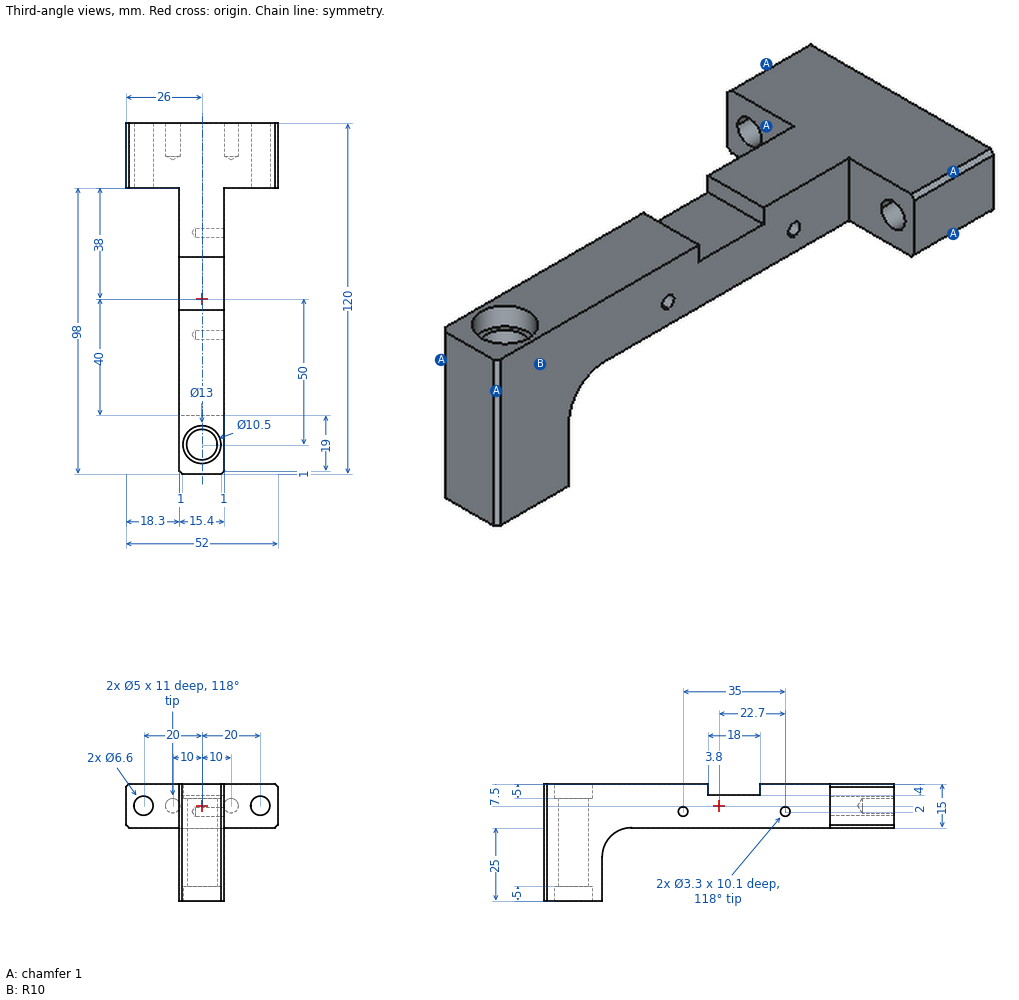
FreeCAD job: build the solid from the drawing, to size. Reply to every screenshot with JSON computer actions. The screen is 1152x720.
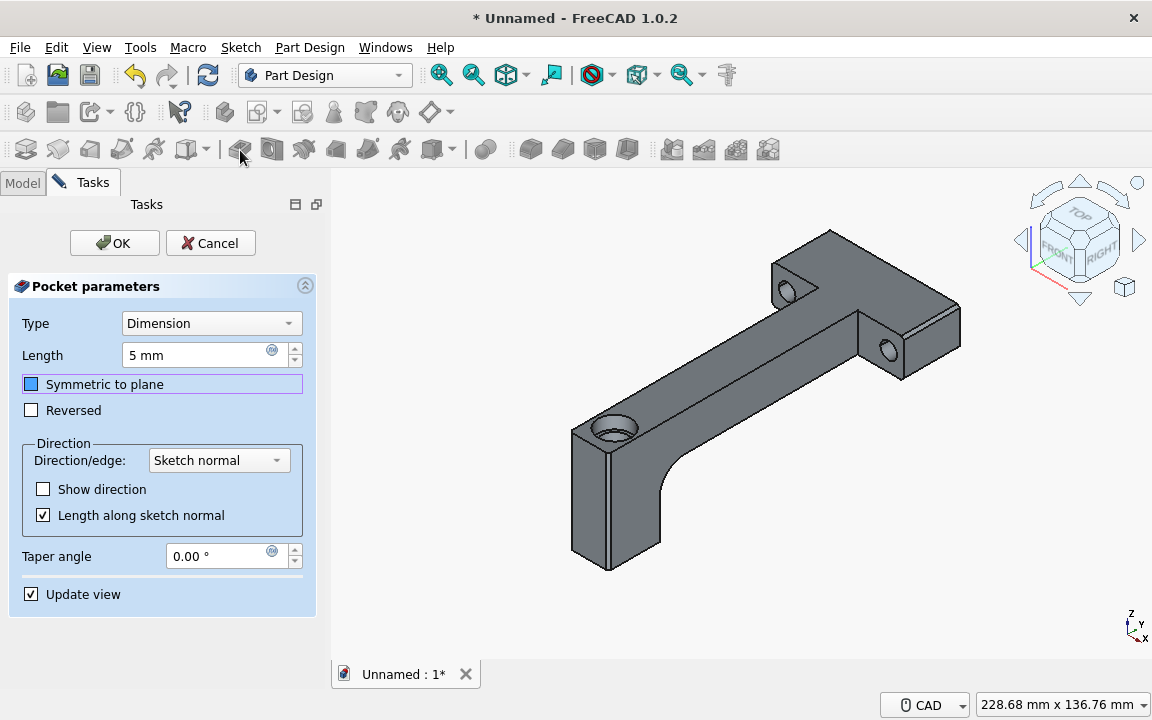
{"action": "left_click", "coordinate": [115, 243]}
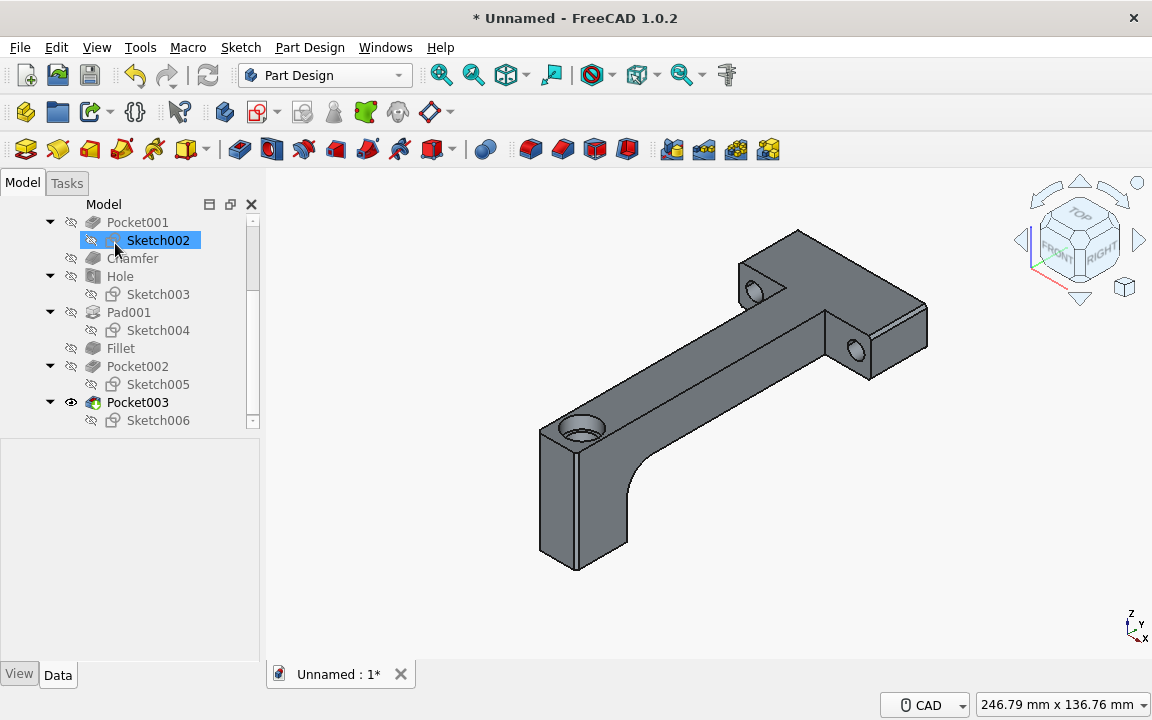
{"action": "scroll", "coordinate": [140, 326], "scroll_direction": "down", "scroll_amount": 3}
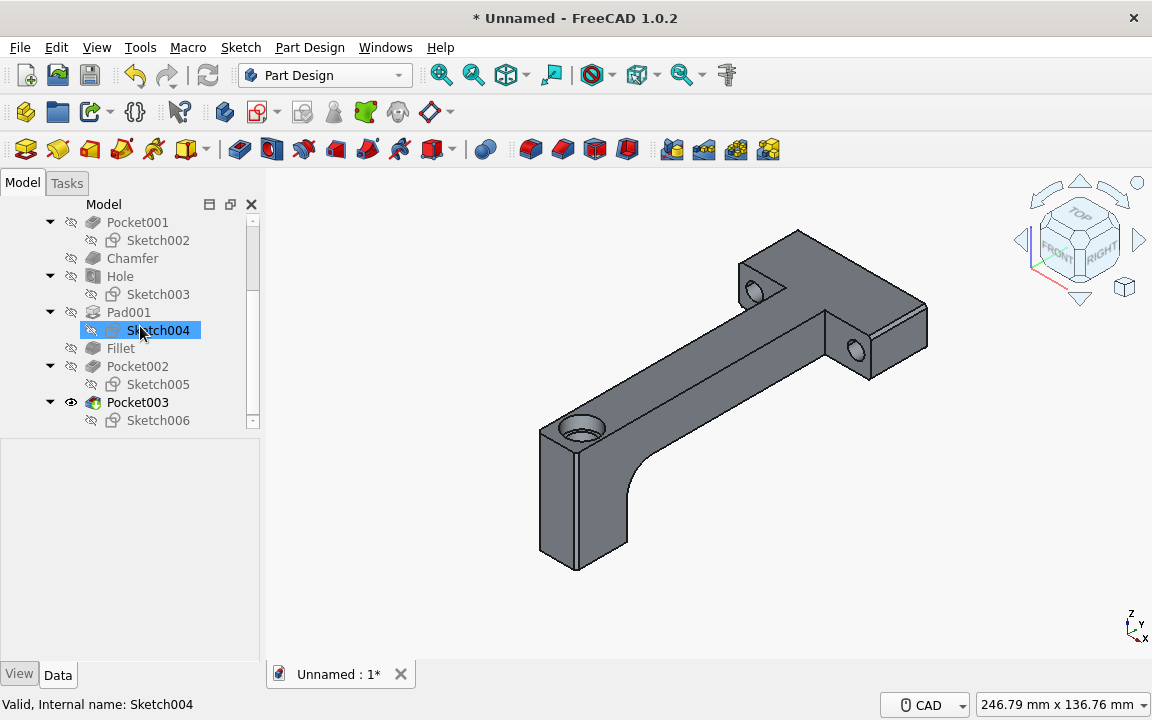
{"action": "scroll", "coordinate": [140, 326], "scroll_direction": "up", "scroll_amount": 15}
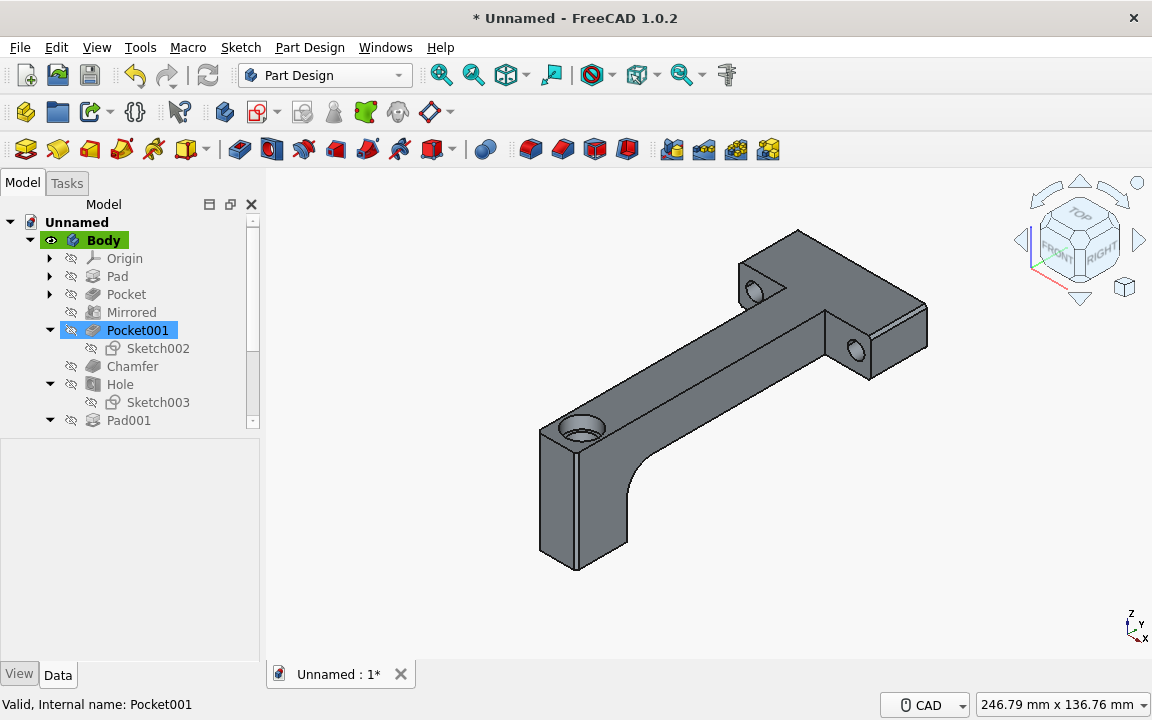
{"action": "left_click", "coordinate": [50, 258]}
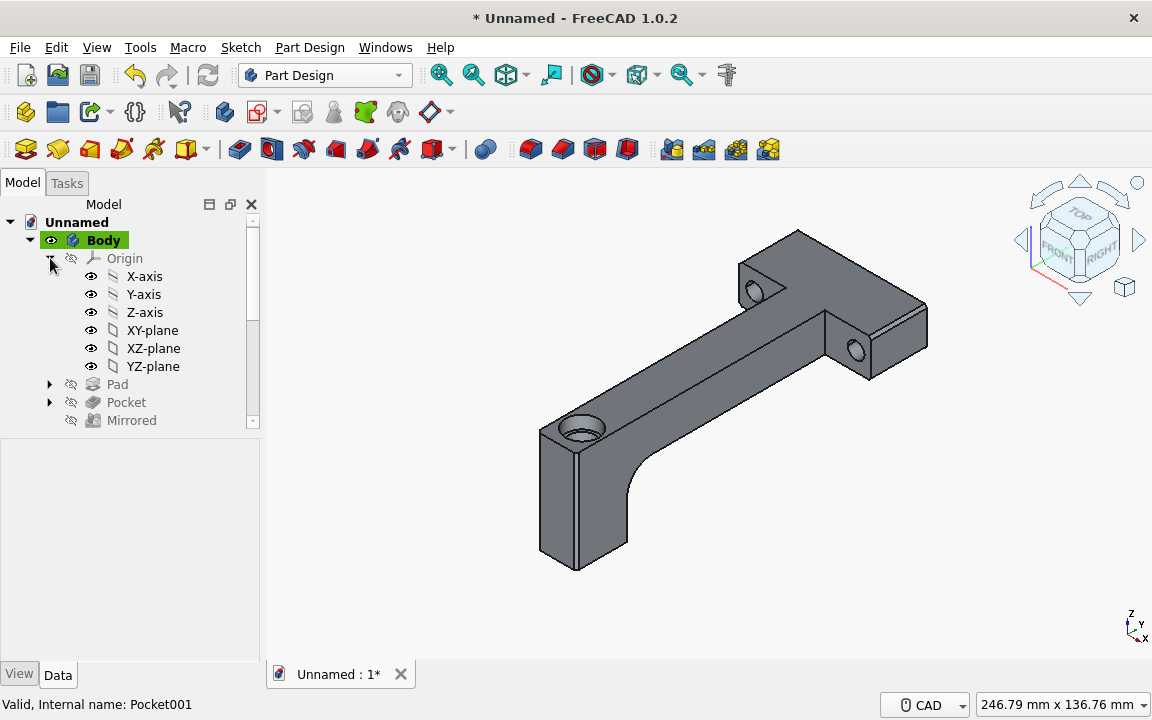
{"action": "left_click", "coordinate": [136, 330]}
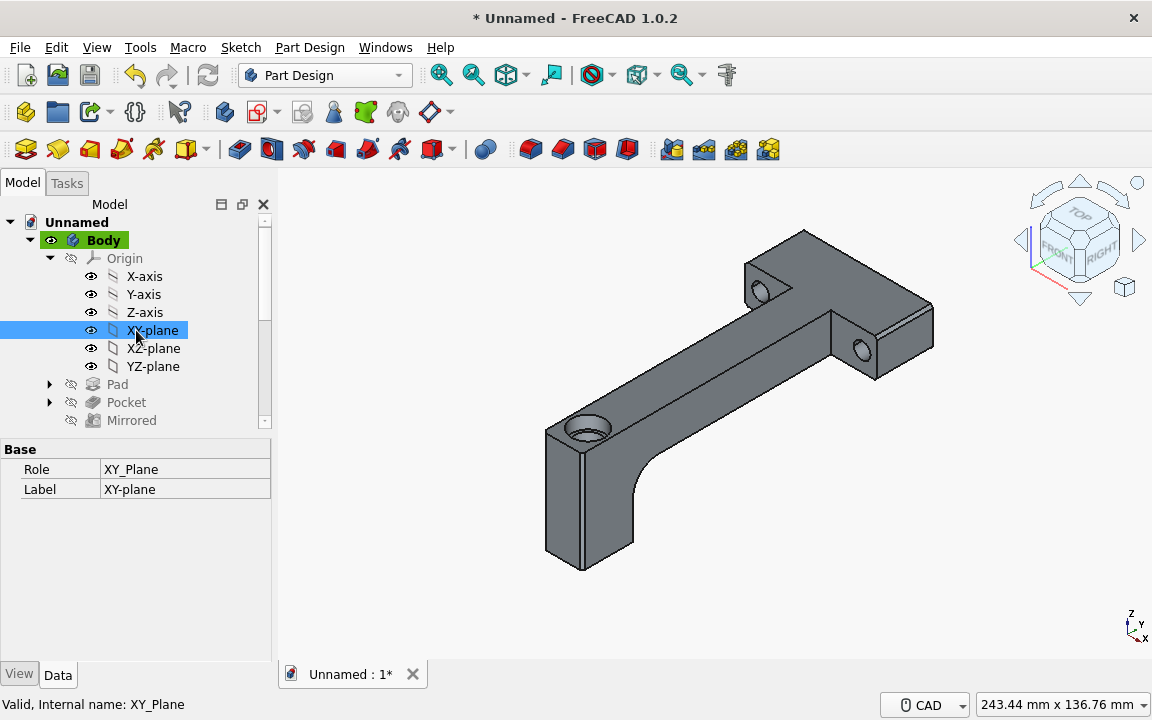
{"action": "left_click", "coordinate": [430, 112]}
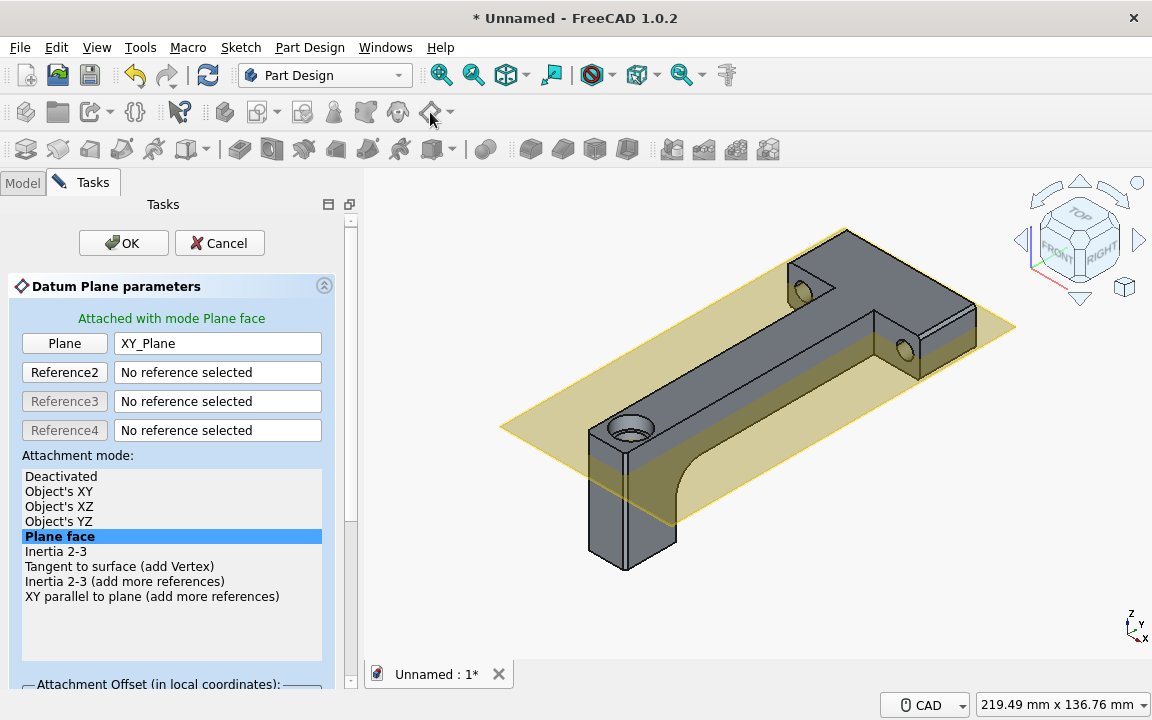
{"action": "scroll", "coordinate": [351, 451], "scroll_direction": "down", "scroll_amount": 3}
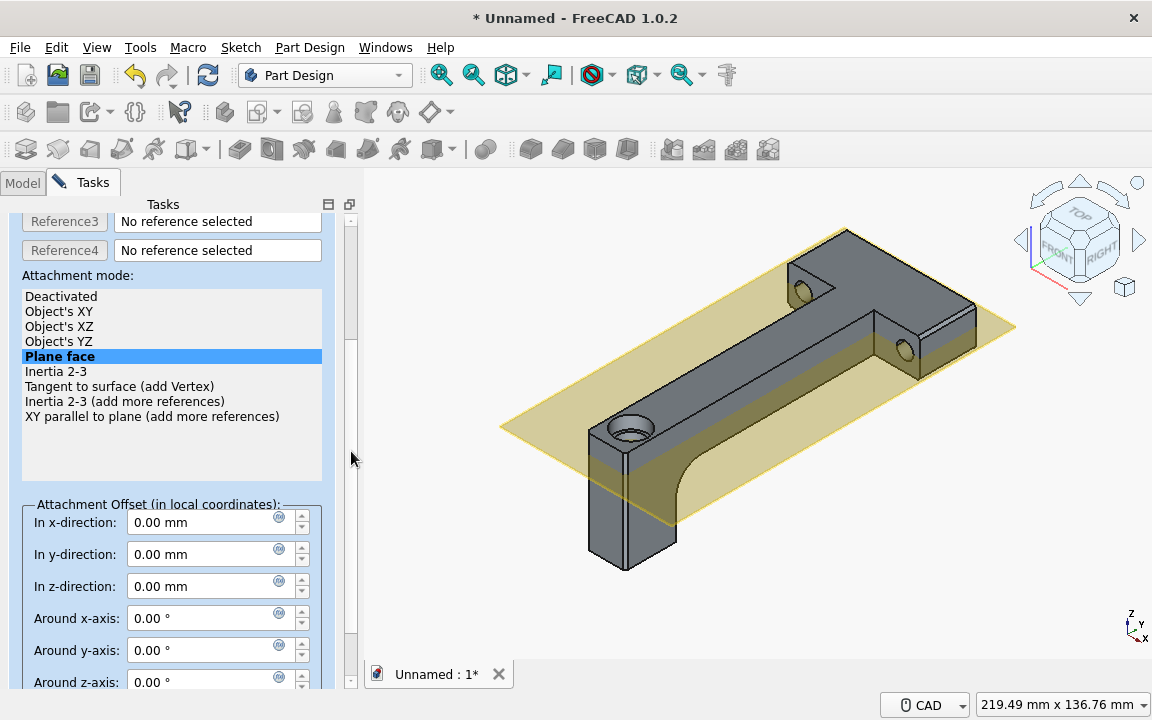
{"action": "triple_click", "coordinate": [210, 586]}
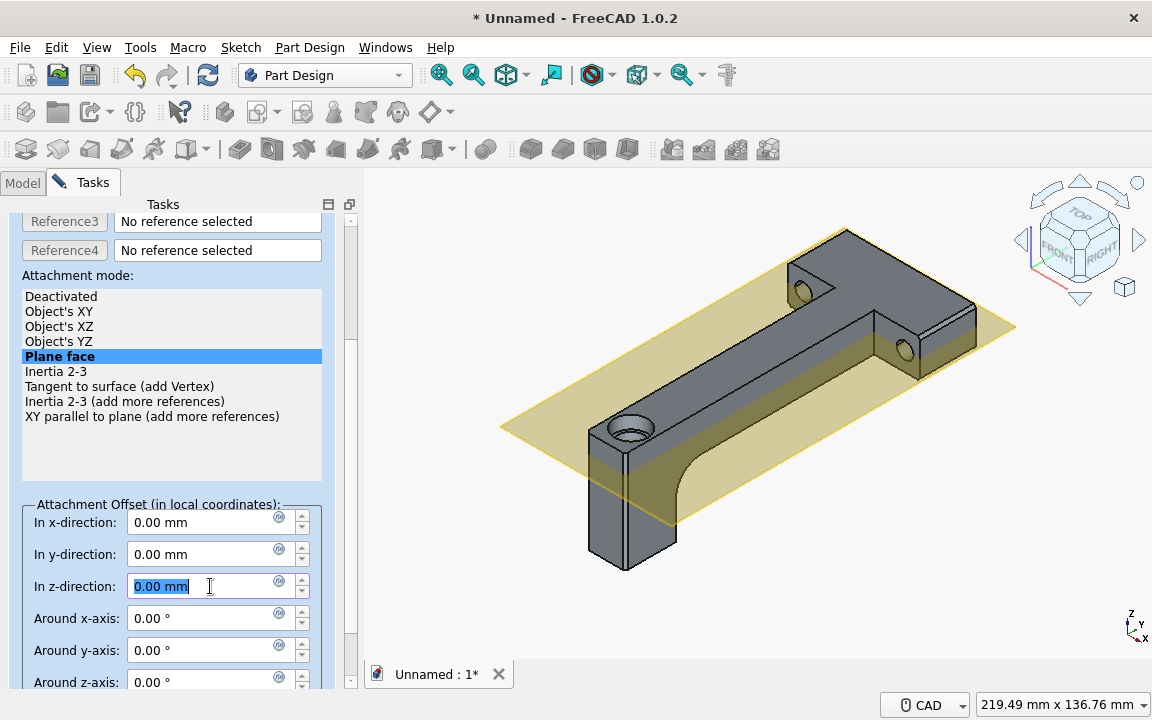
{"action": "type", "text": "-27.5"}
{"action": "key", "text": "Tab"}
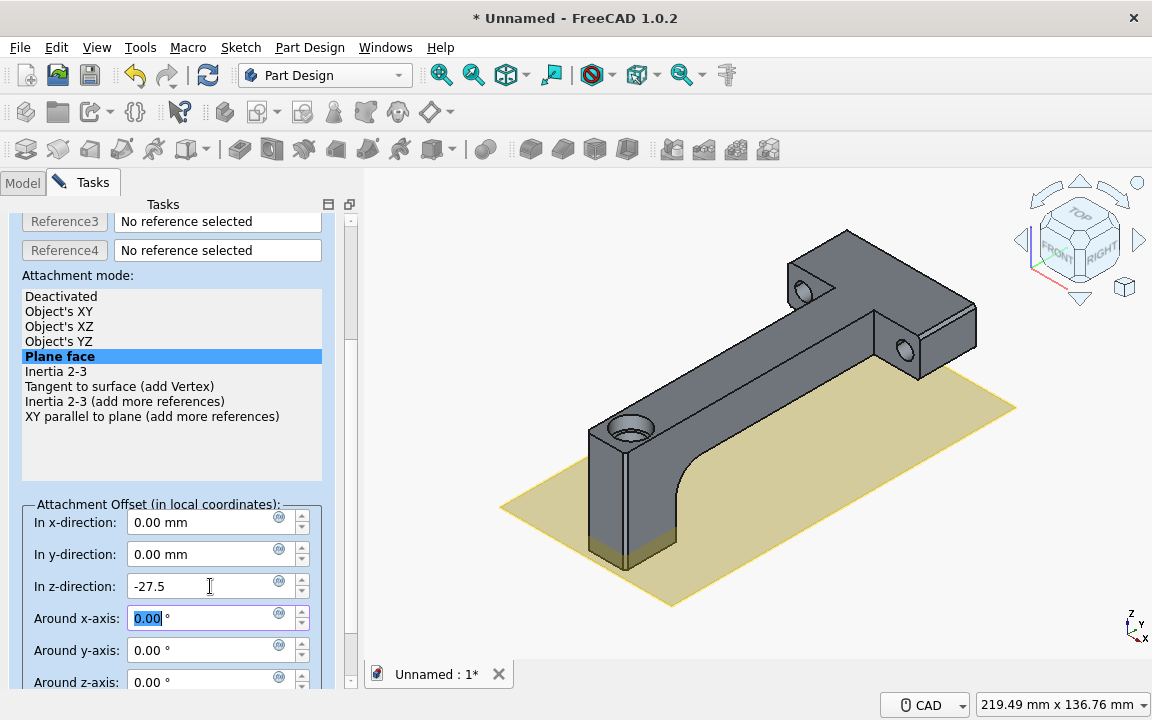
{"action": "scroll", "coordinate": [351, 451], "scroll_direction": "up", "scroll_amount": 4}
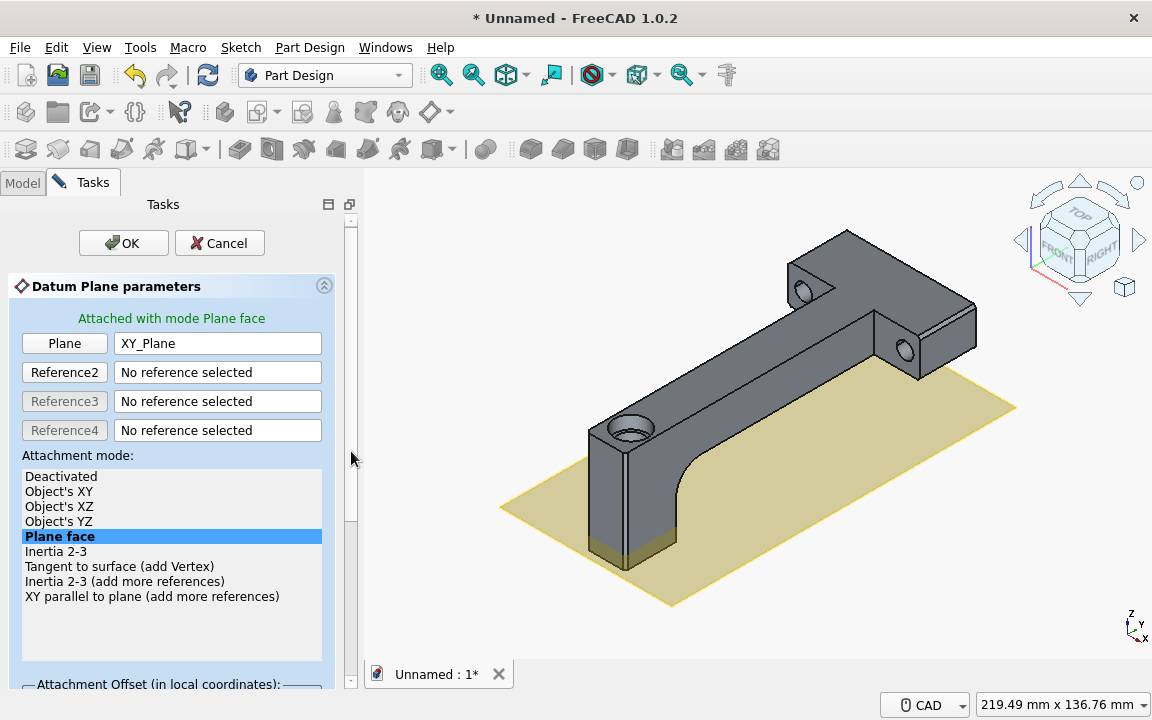
{"action": "left_click", "coordinate": [124, 243]}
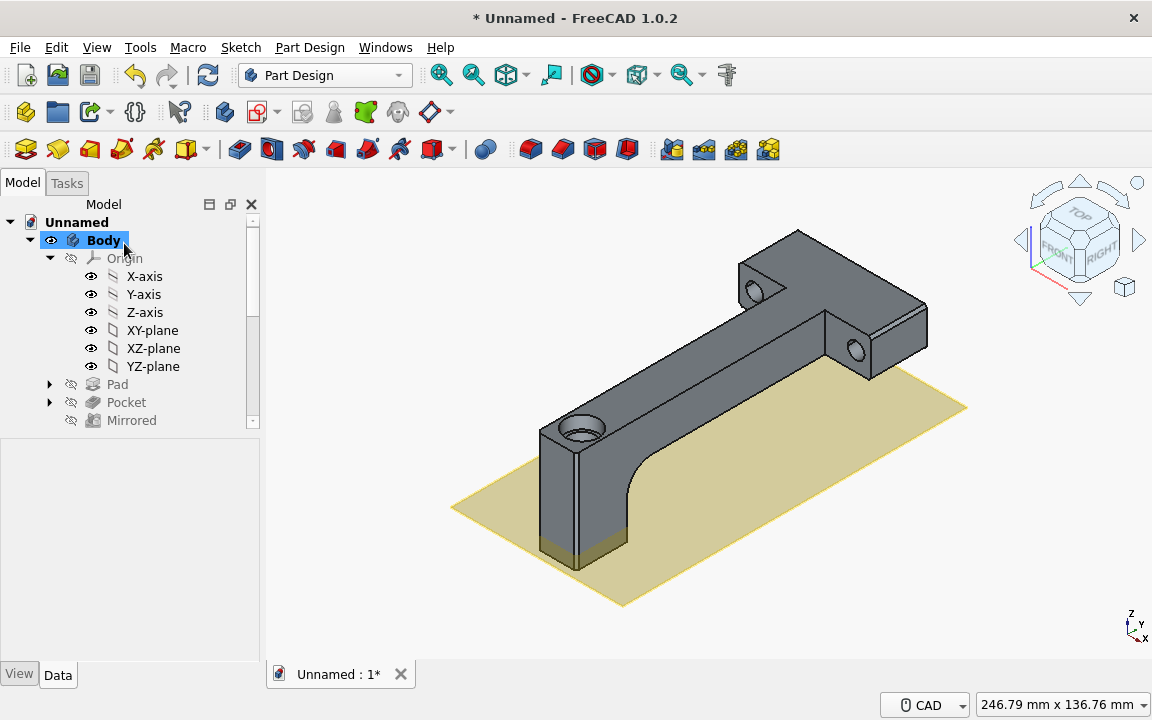
{"action": "scroll", "coordinate": [100, 326], "scroll_direction": "down", "scroll_amount": 3}